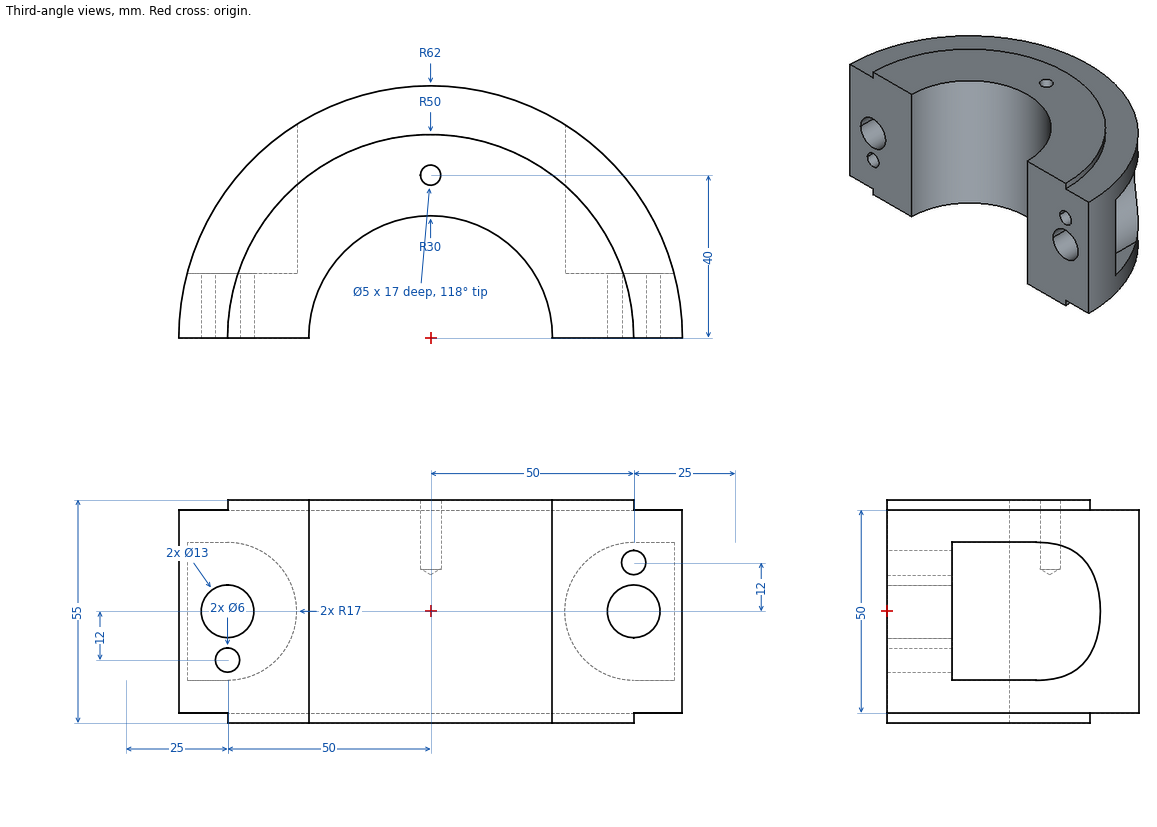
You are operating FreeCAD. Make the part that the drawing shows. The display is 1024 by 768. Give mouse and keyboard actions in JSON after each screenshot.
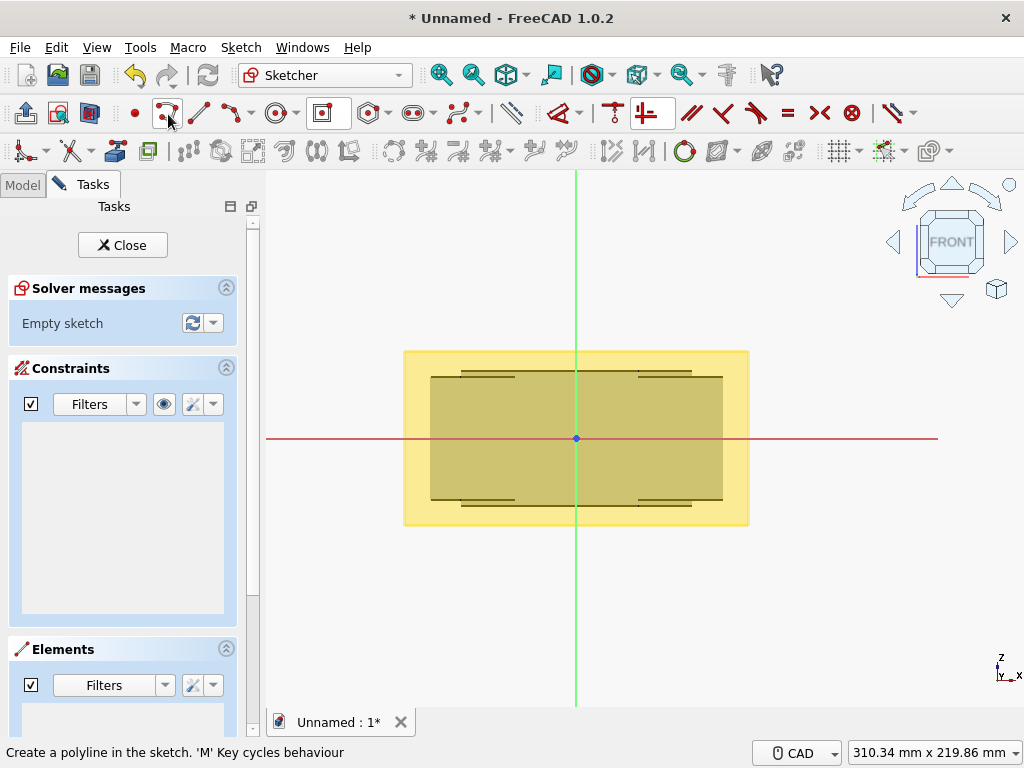
{"action": "left_click", "coordinate": [454, 480]}
{"action": "left_click", "coordinate": [393, 480]}
{"action": "left_click", "coordinate": [393, 397]}
{"action": "left_click", "coordinate": [454, 397]}
{"action": "right_click", "coordinate": [454, 397]}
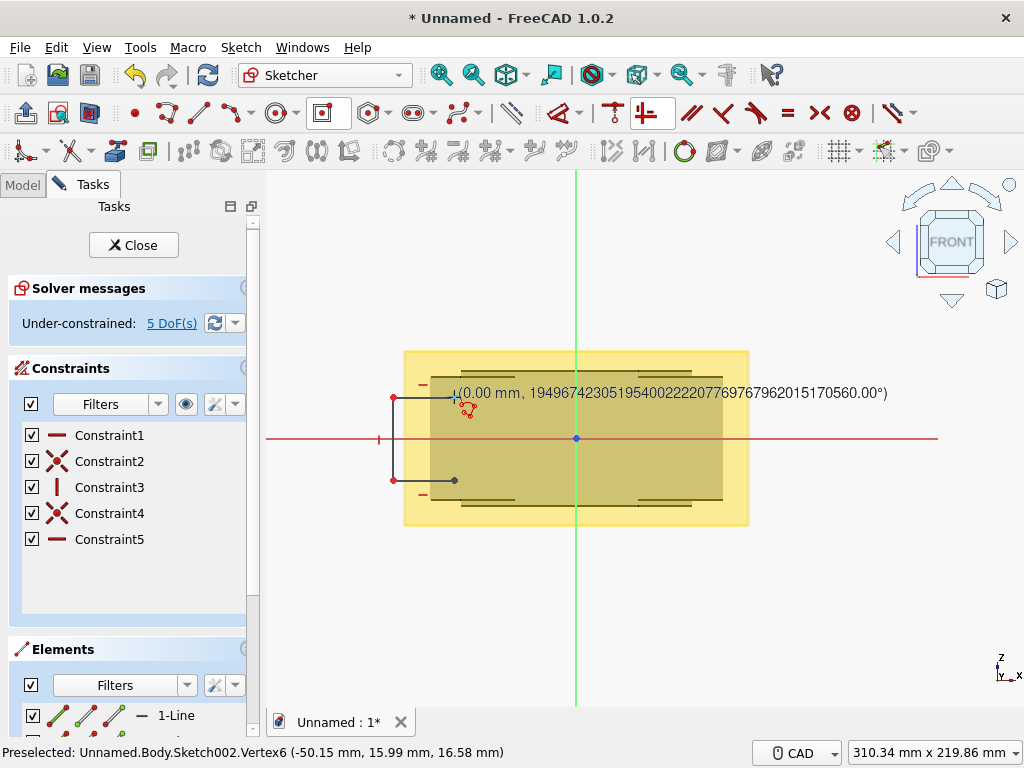
{"action": "left_click", "coordinate": [232, 114]}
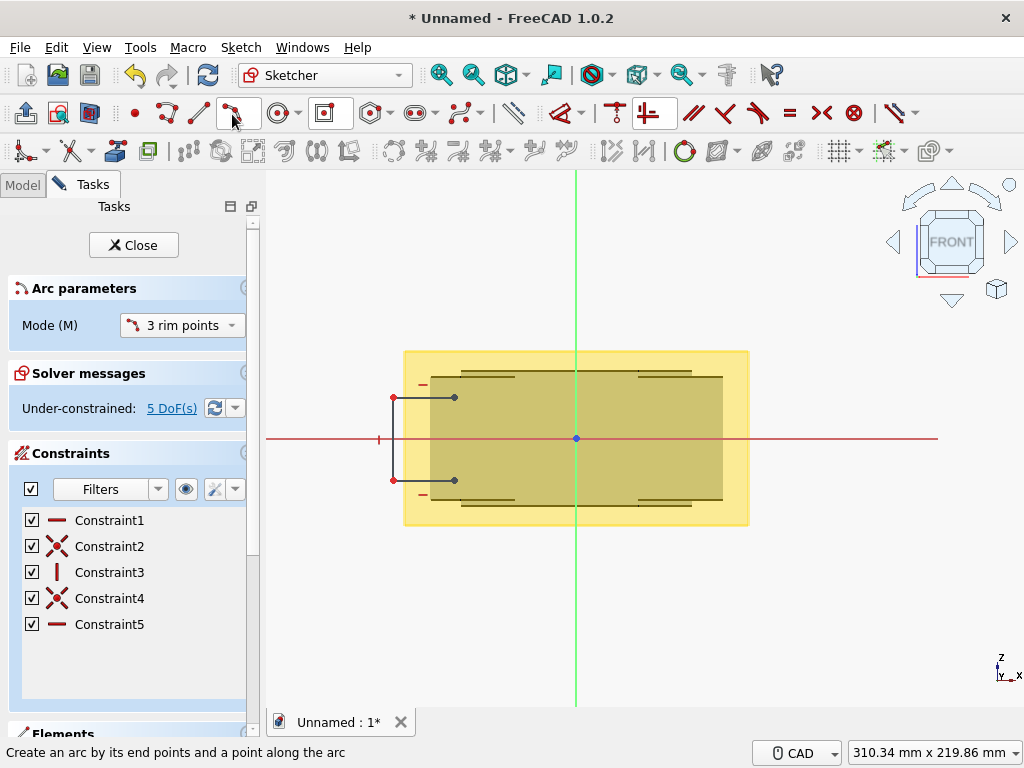
{"action": "left_click", "coordinate": [454, 398]}
{"action": "left_click", "coordinate": [454, 481]}
{"action": "left_click", "coordinate": [488, 463]}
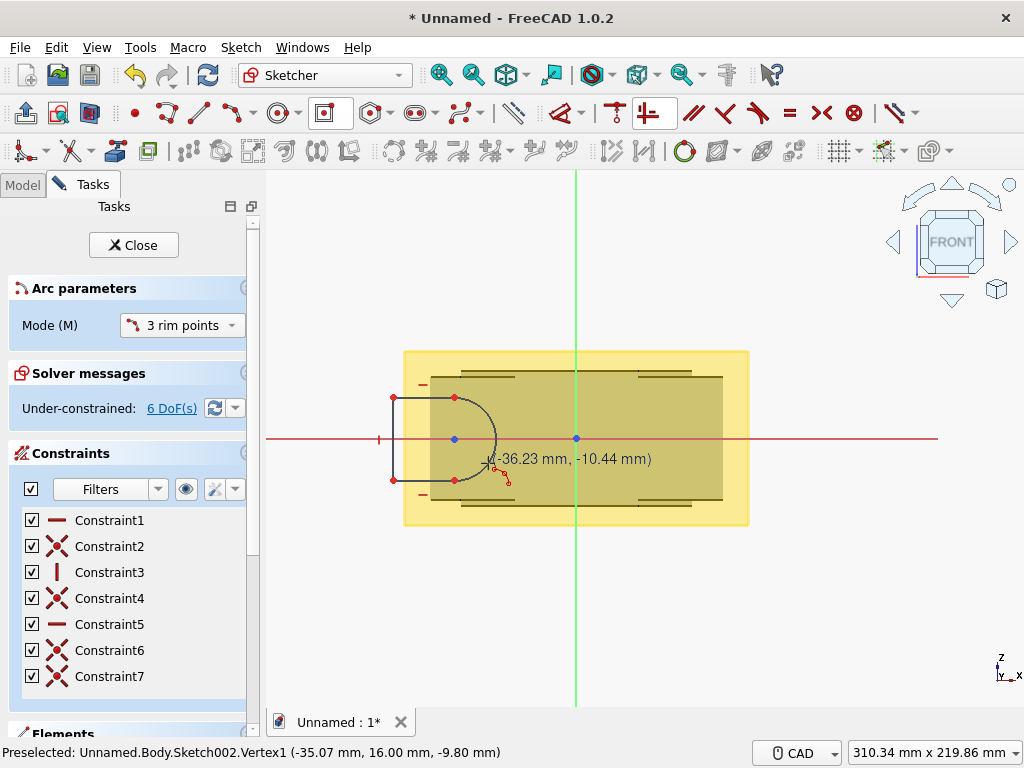
{"action": "key", "text": "g m"}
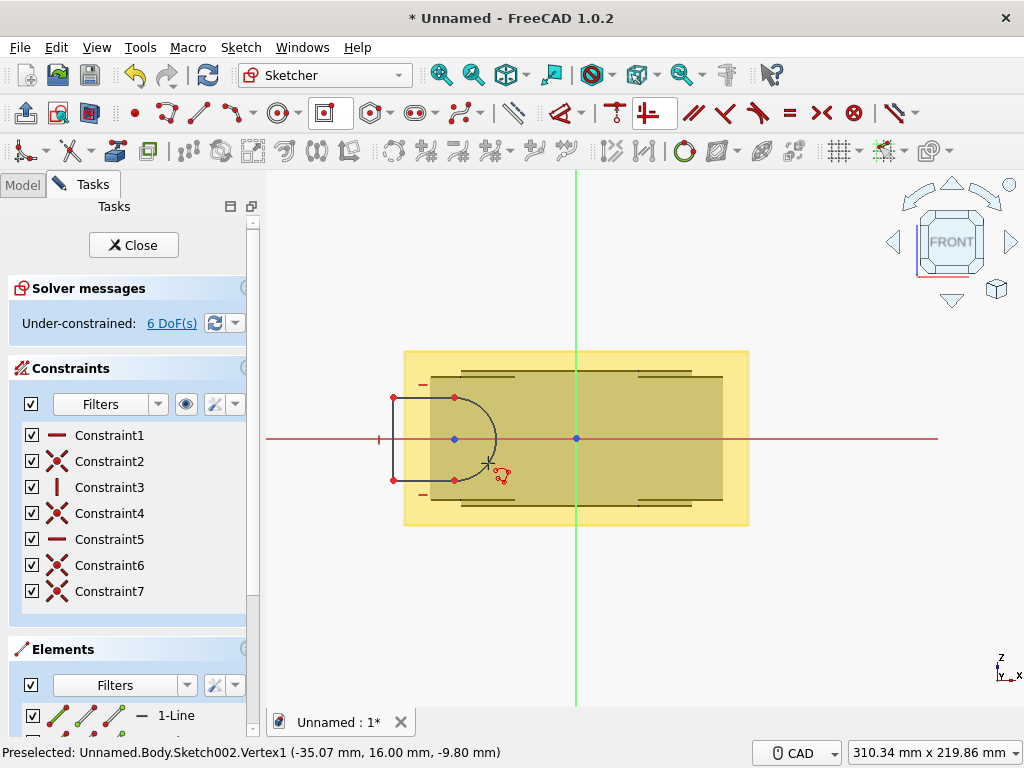
{"action": "left_click", "coordinate": [699, 397]}
{"action": "left_click", "coordinate": [760, 397]}
{"action": "left_click", "coordinate": [760, 480]}
{"action": "left_click", "coordinate": [699, 480]}
{"action": "right_click", "coordinate": [699, 480]}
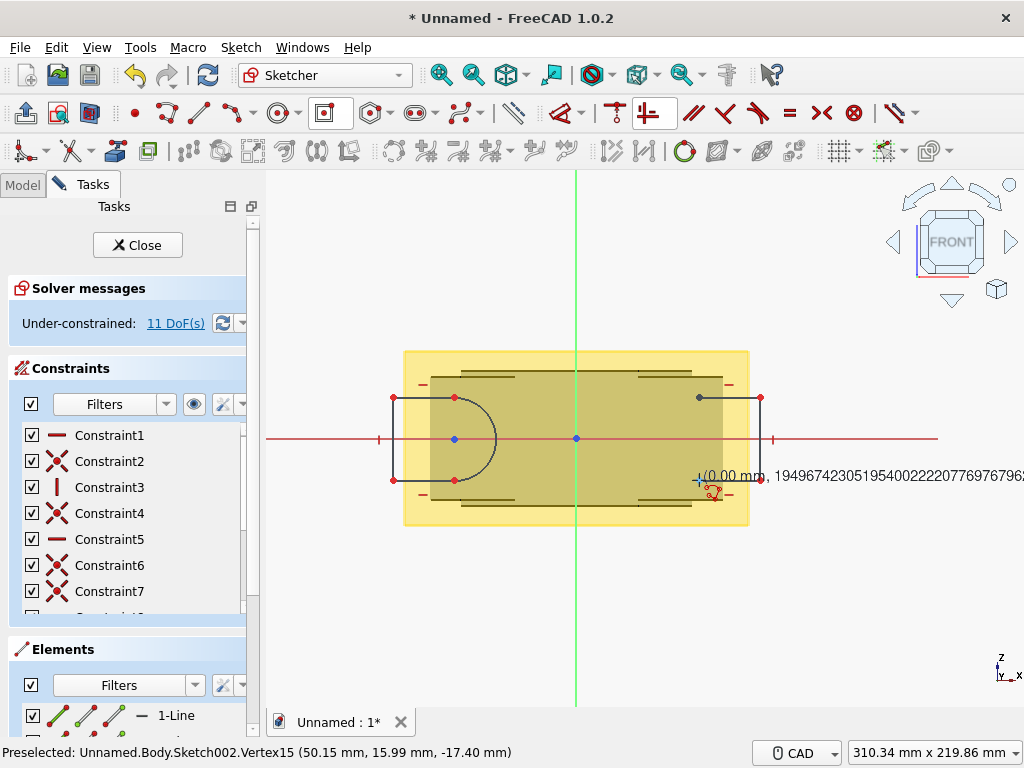
{"action": "key", "text": "g 3 a"}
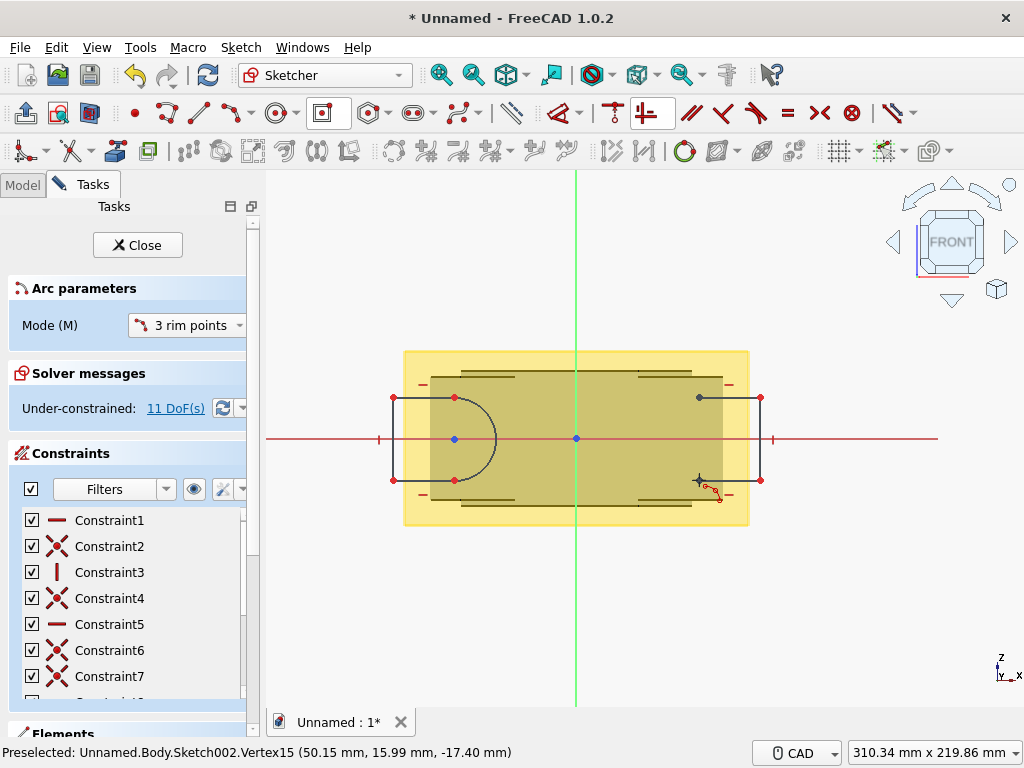
{"action": "left_click", "coordinate": [699, 481]}
{"action": "left_click", "coordinate": [699, 398]}
{"action": "left_click", "coordinate": [665, 414]}
{"action": "key", "text": "Escape"}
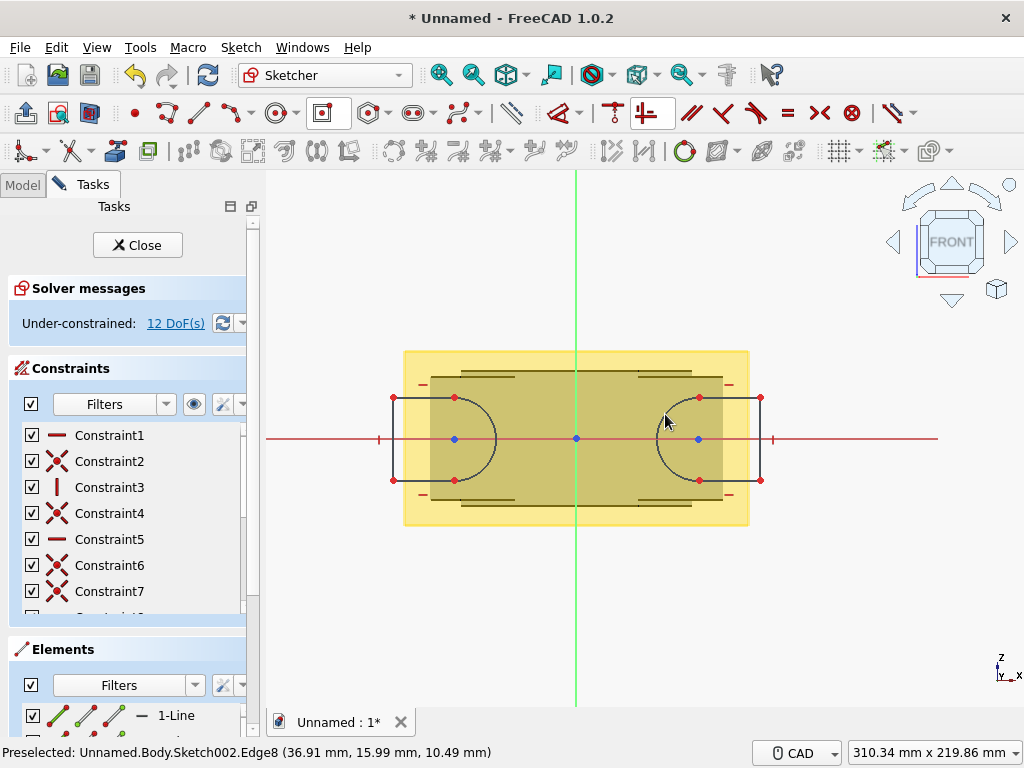
{"action": "left_click", "coordinate": [436, 481]}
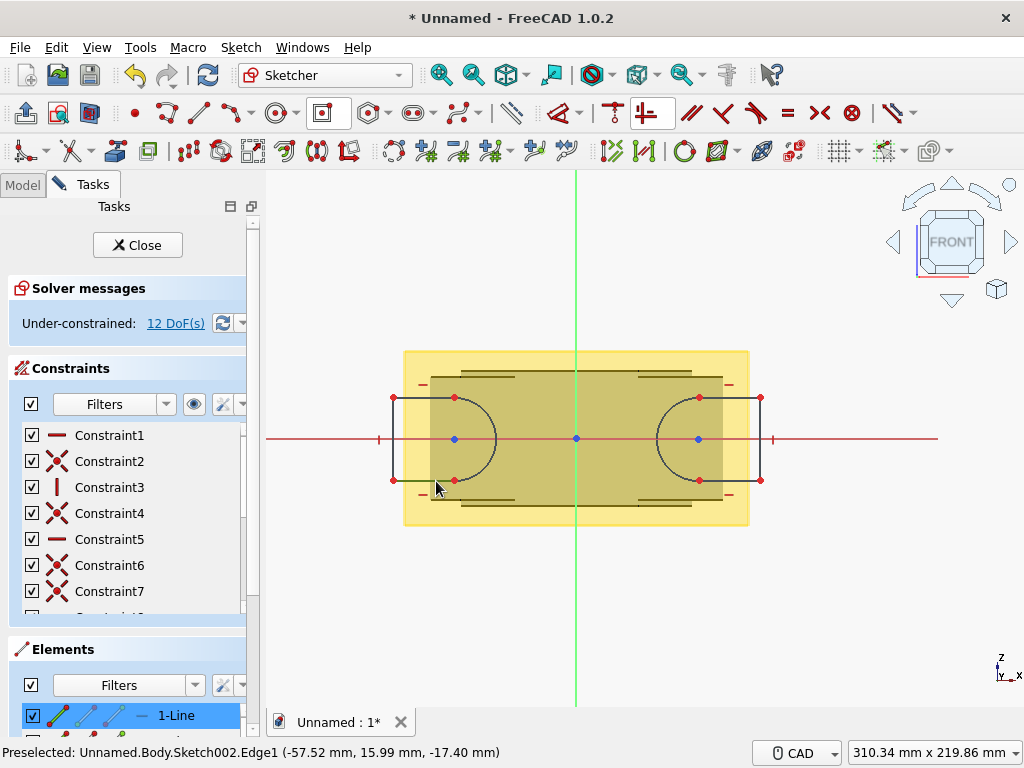
{"action": "left_click", "coordinate": [488, 464]}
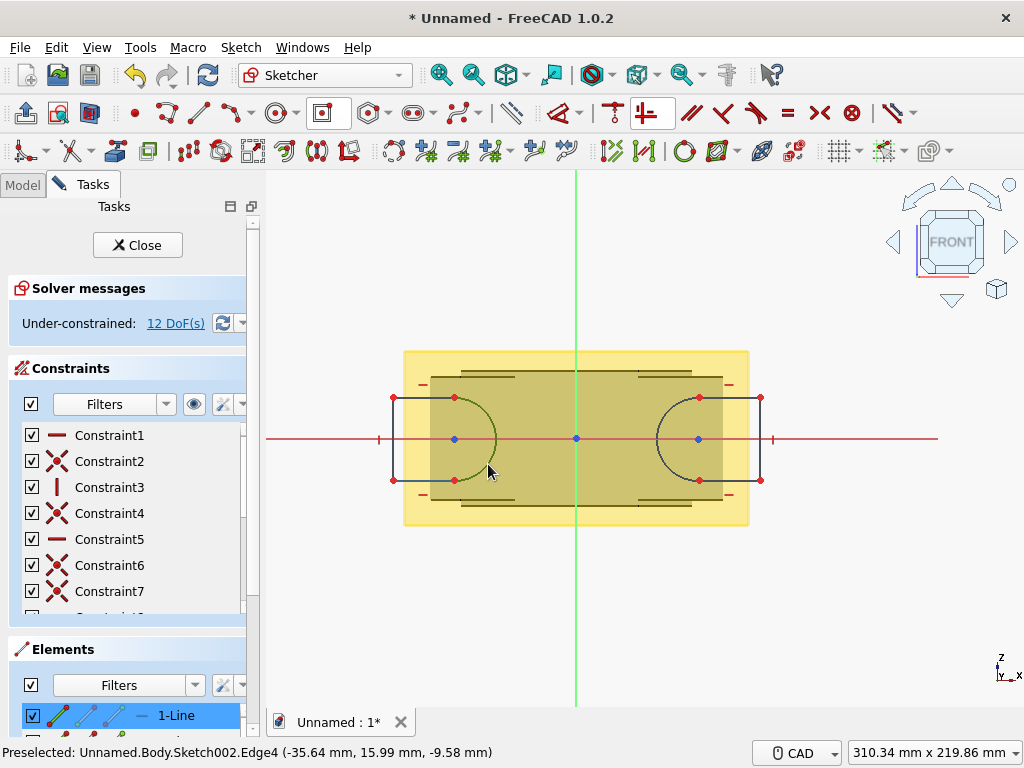
{"action": "left_click", "coordinate": [756, 114]}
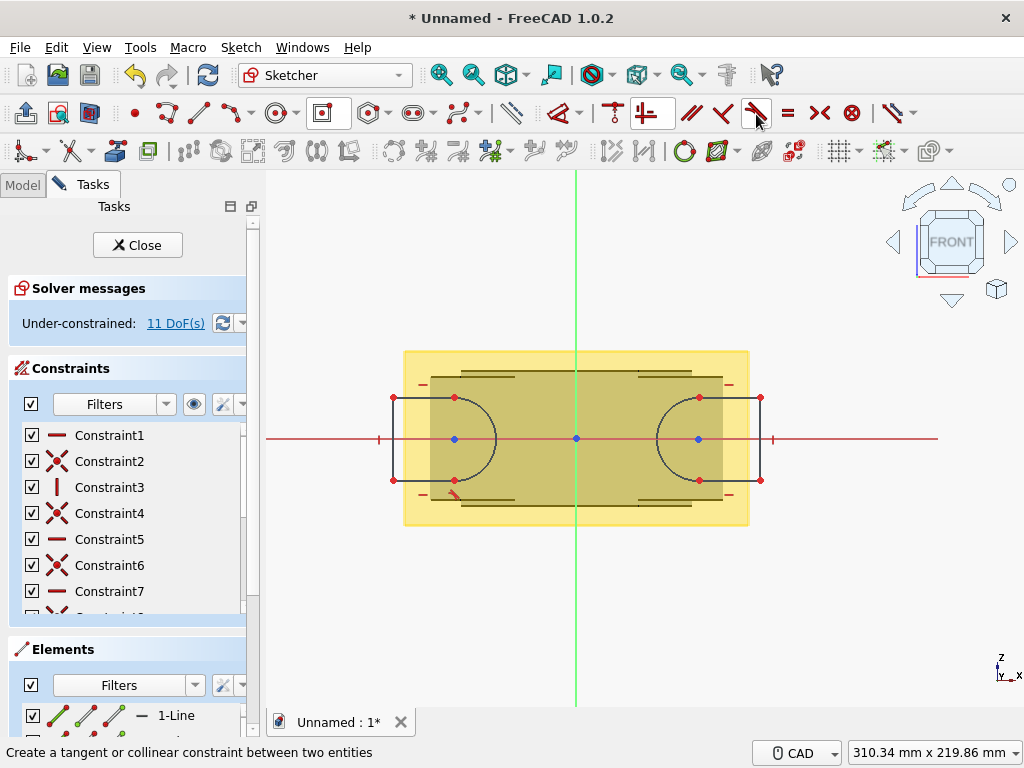
{"action": "left_click", "coordinate": [411, 398]}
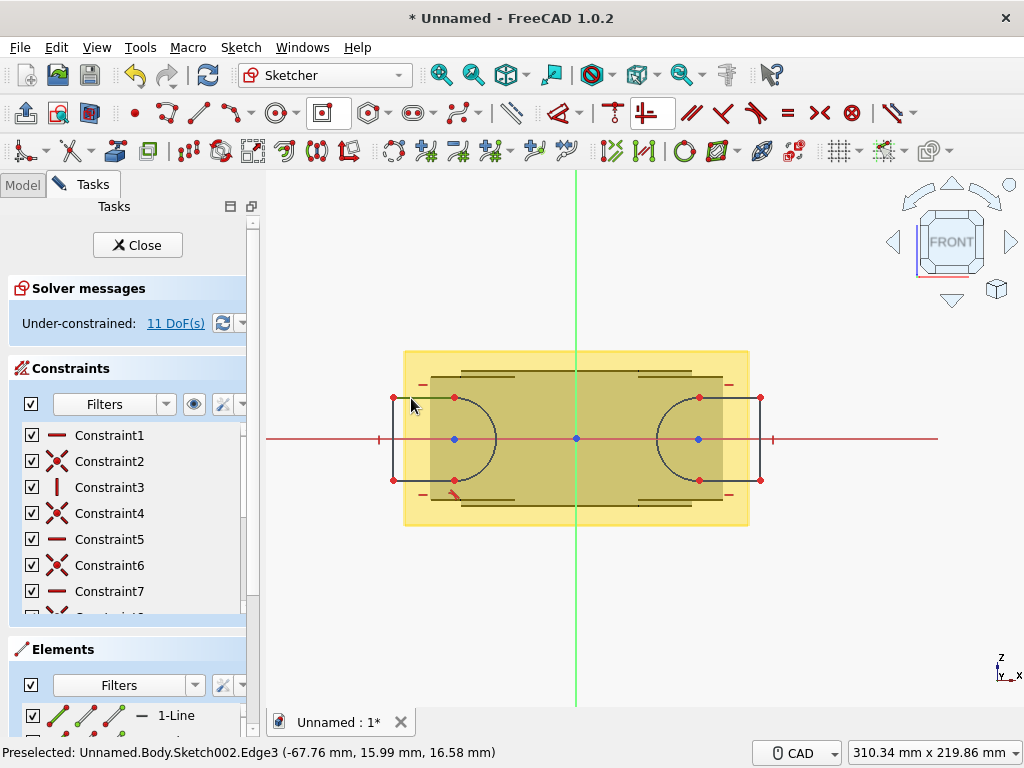
{"action": "left_click", "coordinate": [488, 464]}